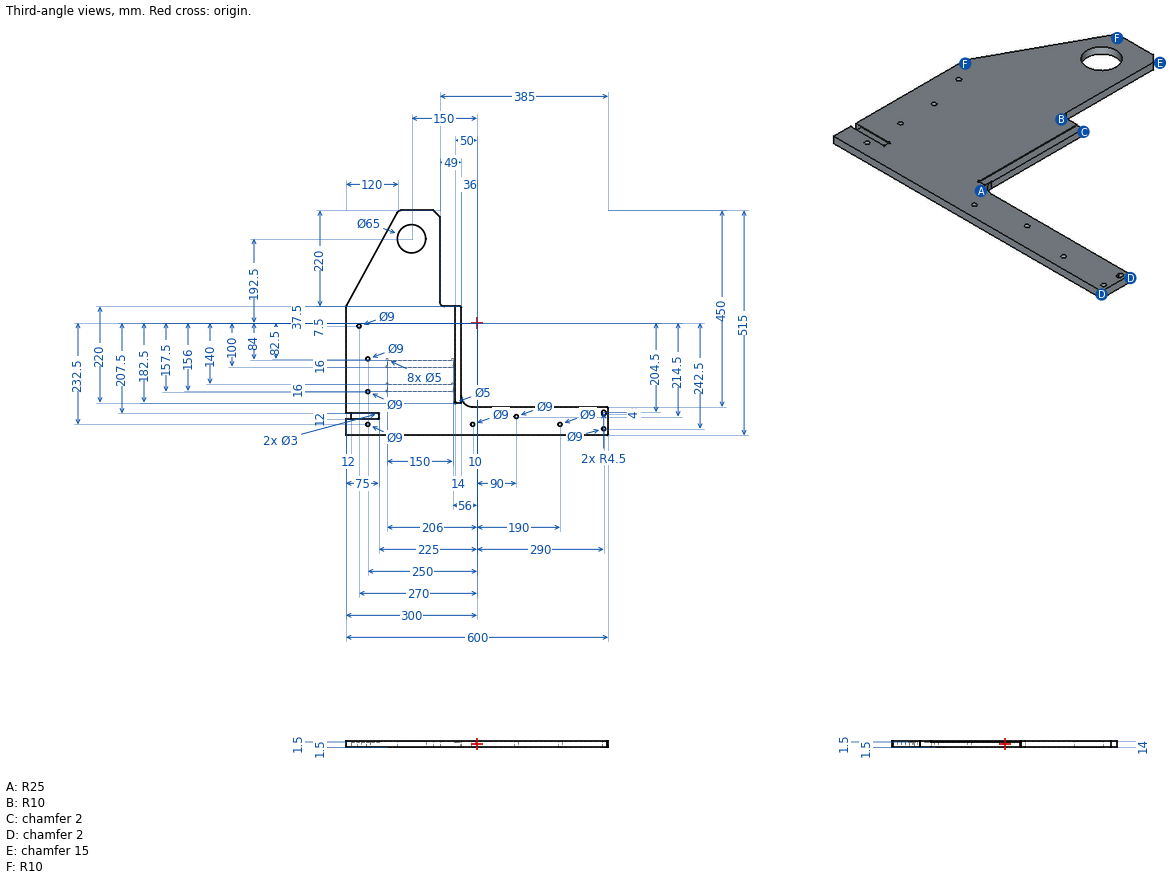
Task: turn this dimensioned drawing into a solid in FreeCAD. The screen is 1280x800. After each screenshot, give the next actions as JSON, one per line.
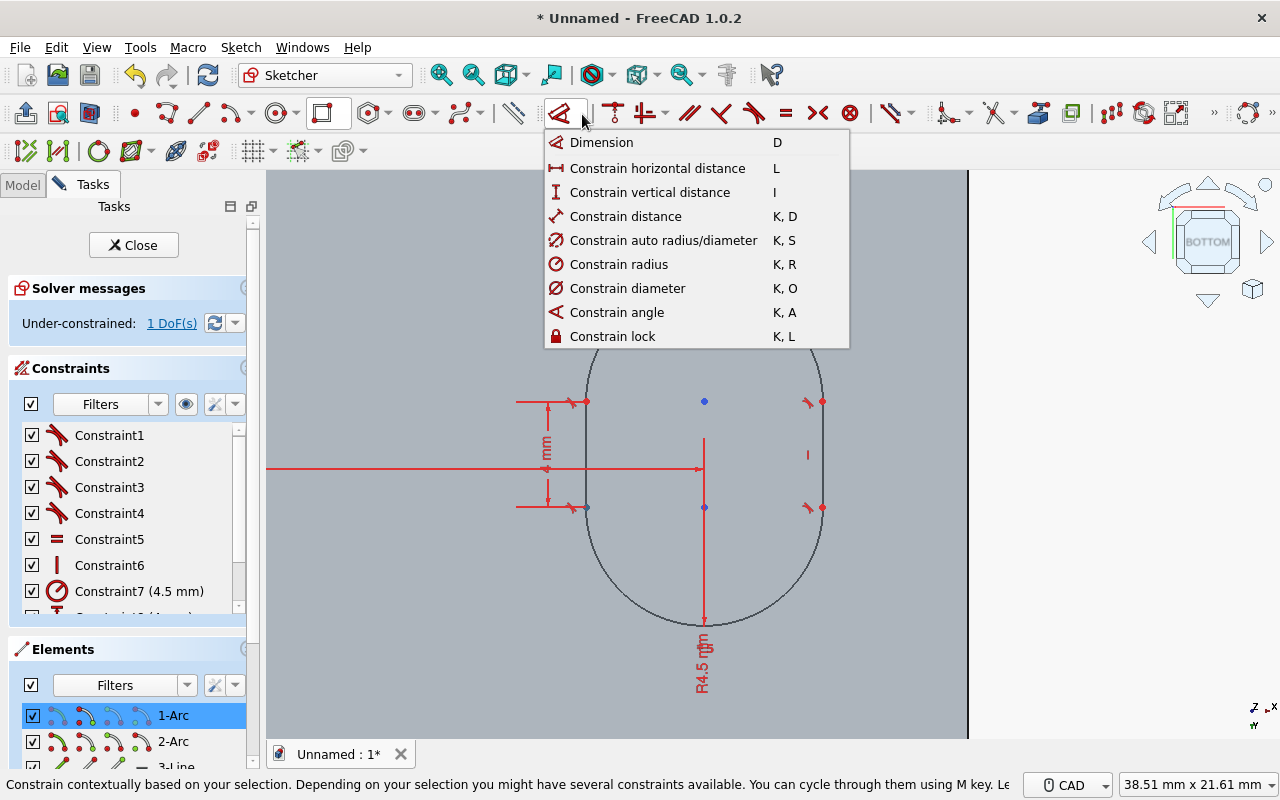
{"action": "left_click", "coordinate": [697, 192]}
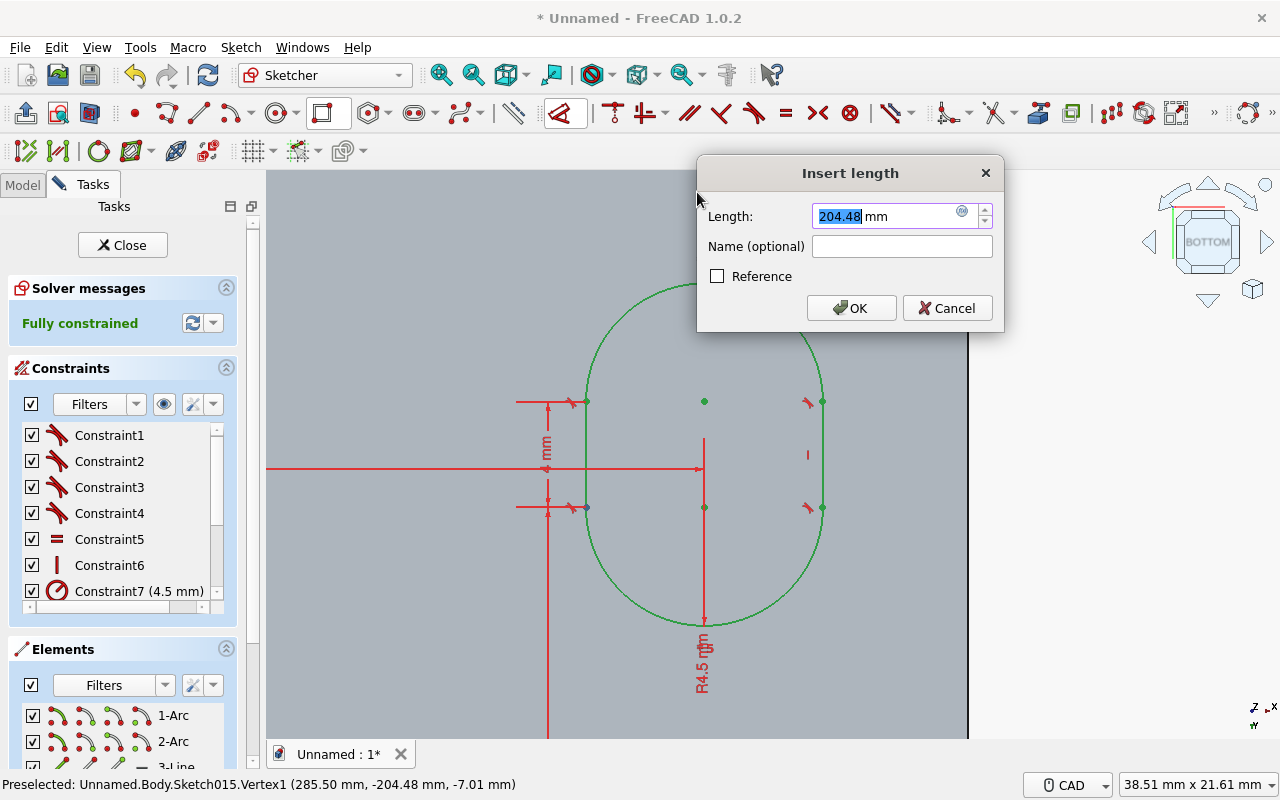
{"action": "type", "text": "204.5"}
{"action": "key", "text": "Return"}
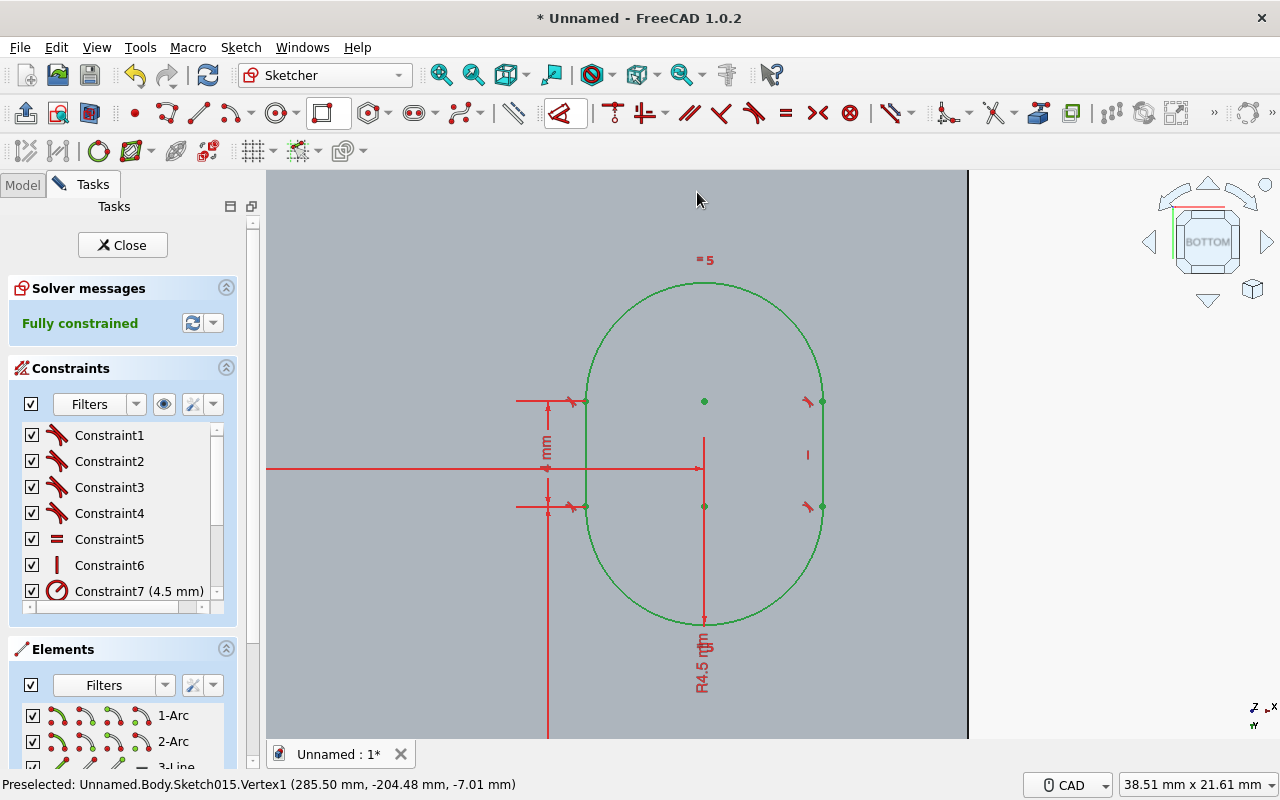
{"action": "left_click", "coordinate": [123, 245]}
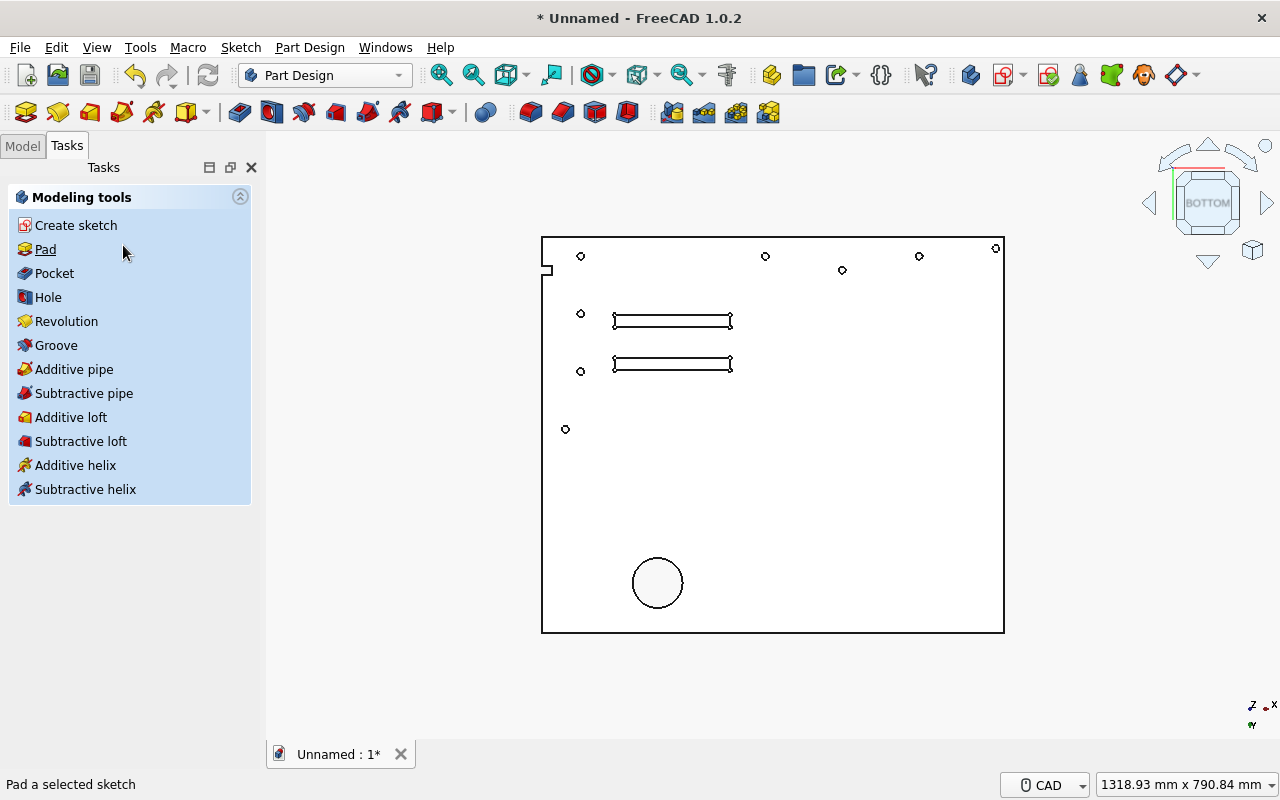
{"action": "left_click", "coordinate": [240, 112]}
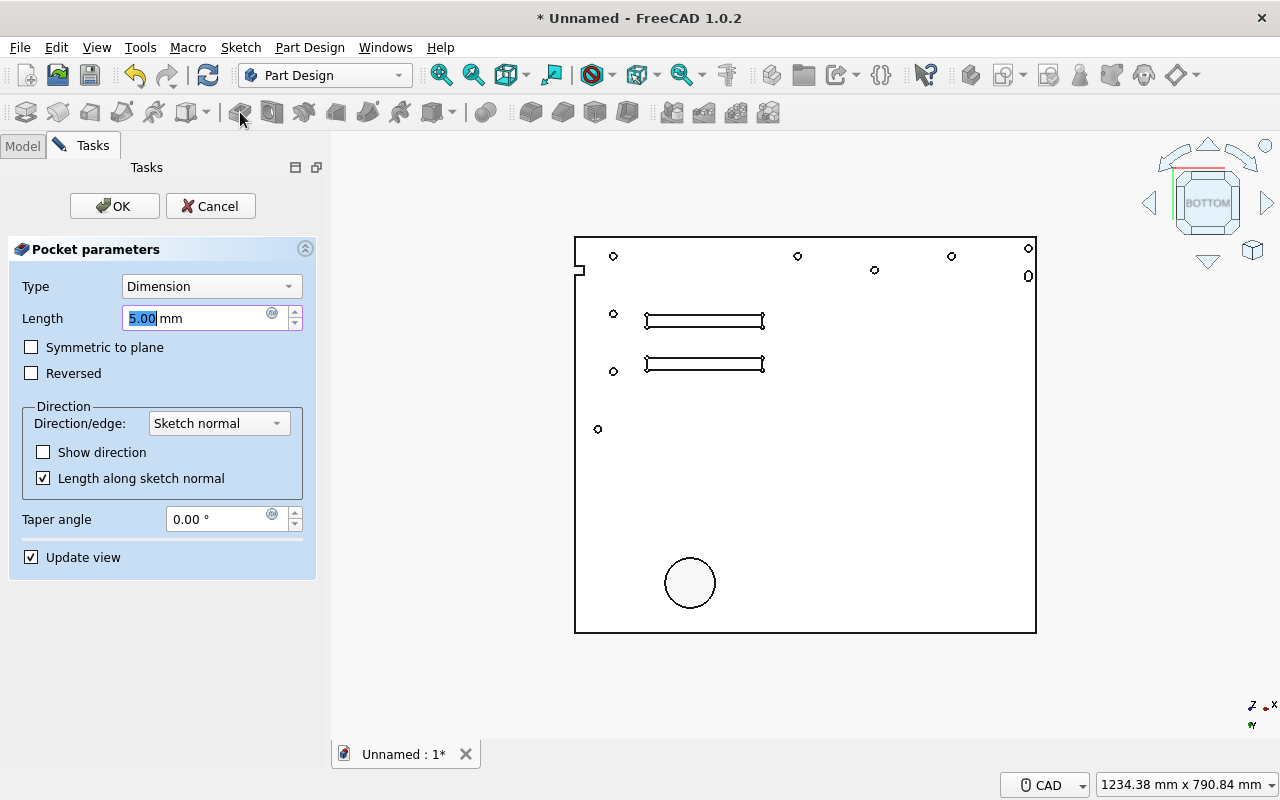
{"action": "left_click", "coordinate": [212, 286]}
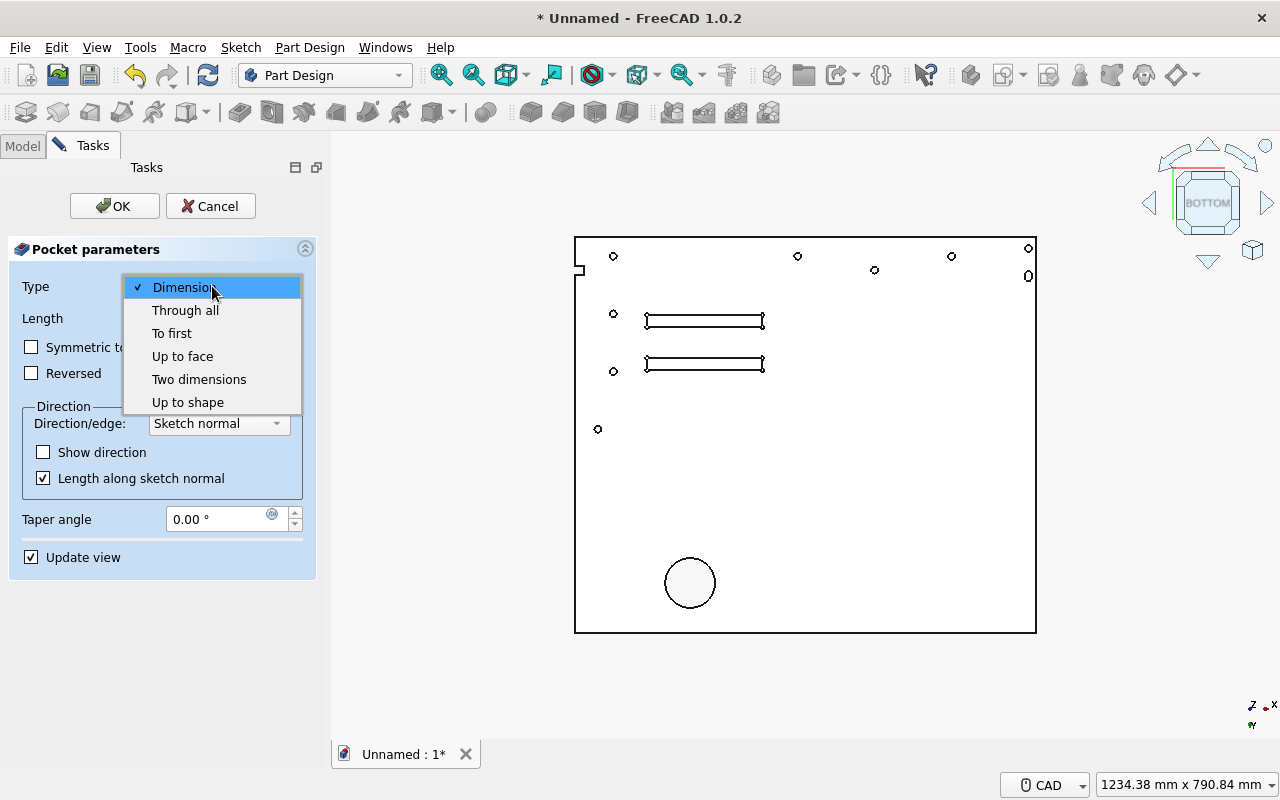
{"action": "left_click", "coordinate": [212, 334]}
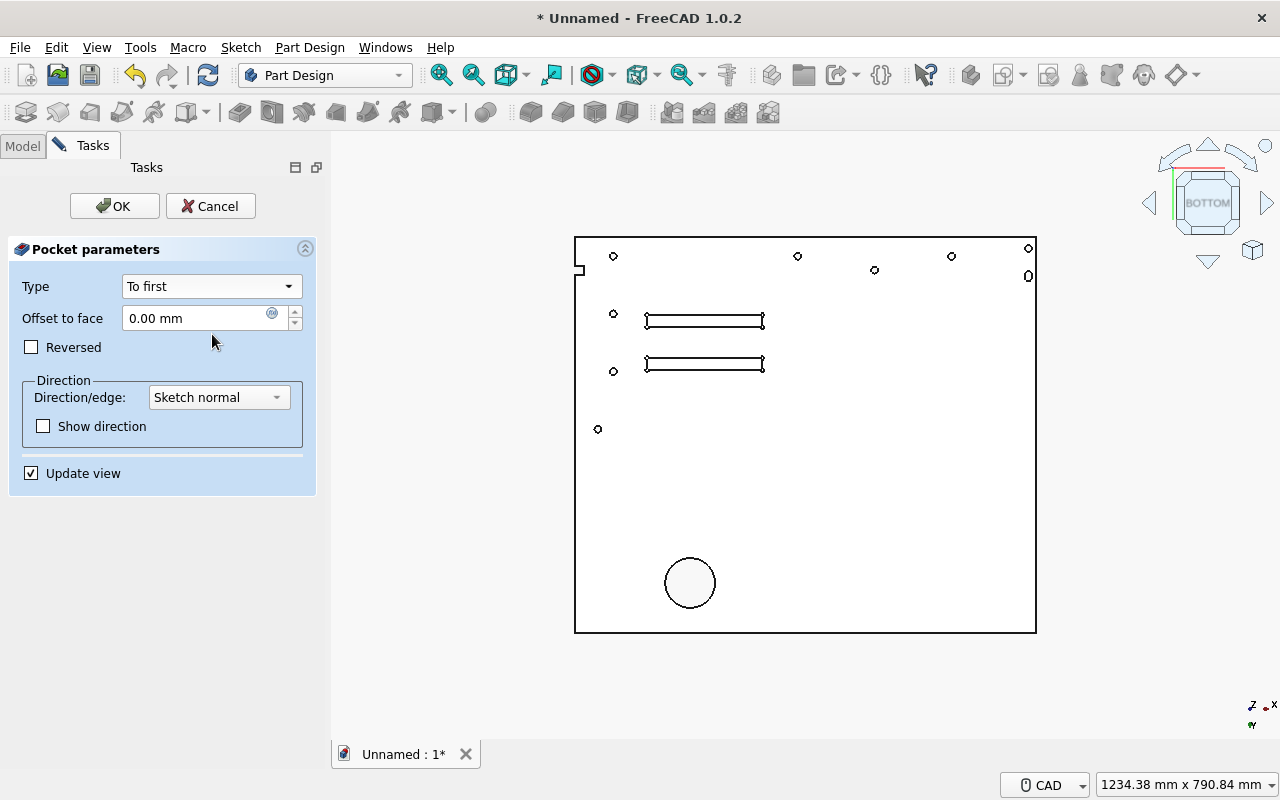
{"action": "left_click", "coordinate": [115, 206]}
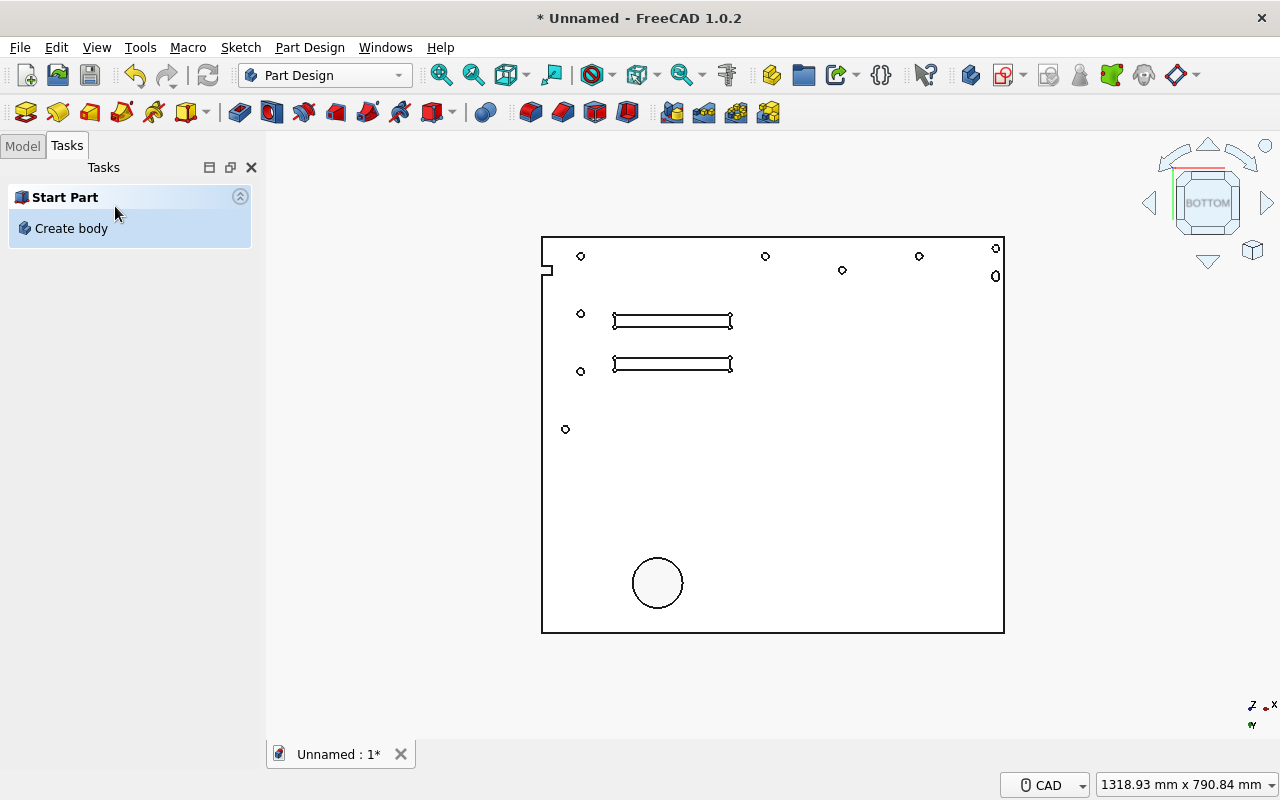
{"action": "left_click", "coordinate": [839, 491]}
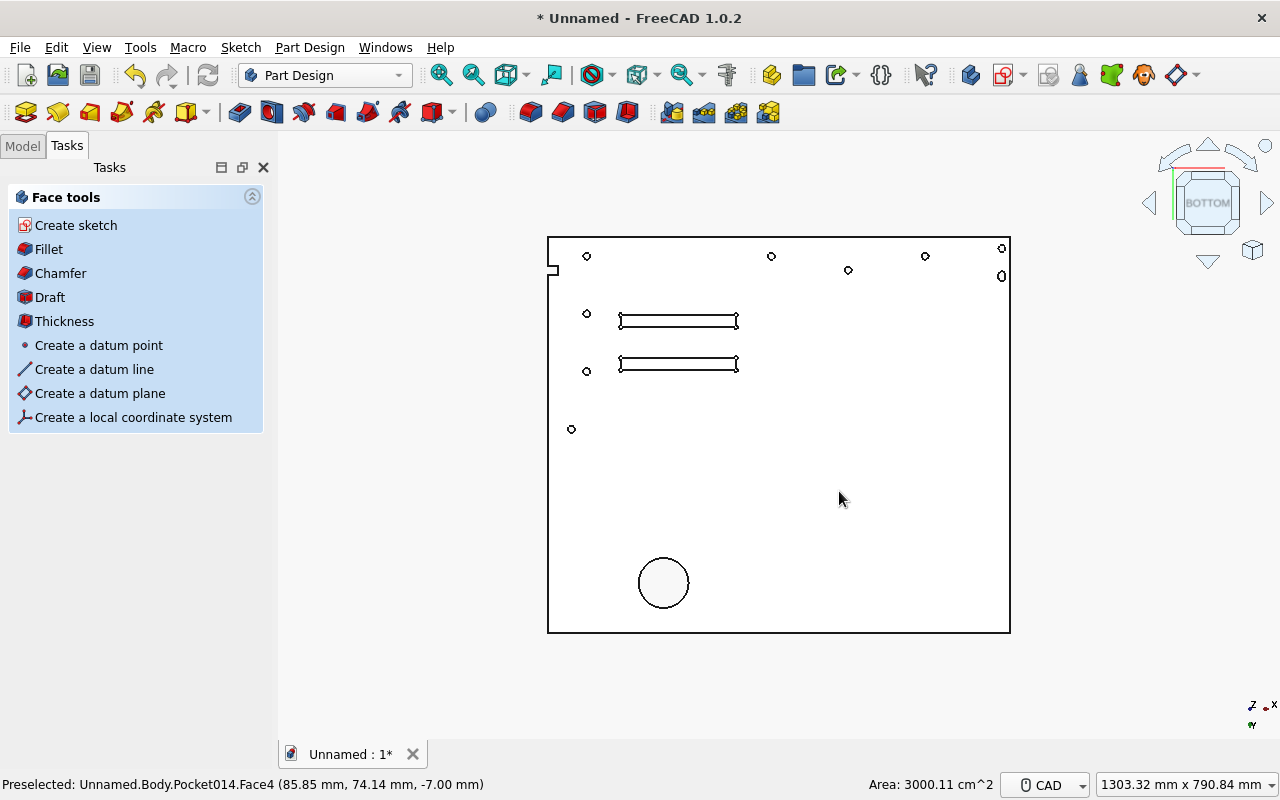
{"action": "left_click", "coordinate": [1004, 76]}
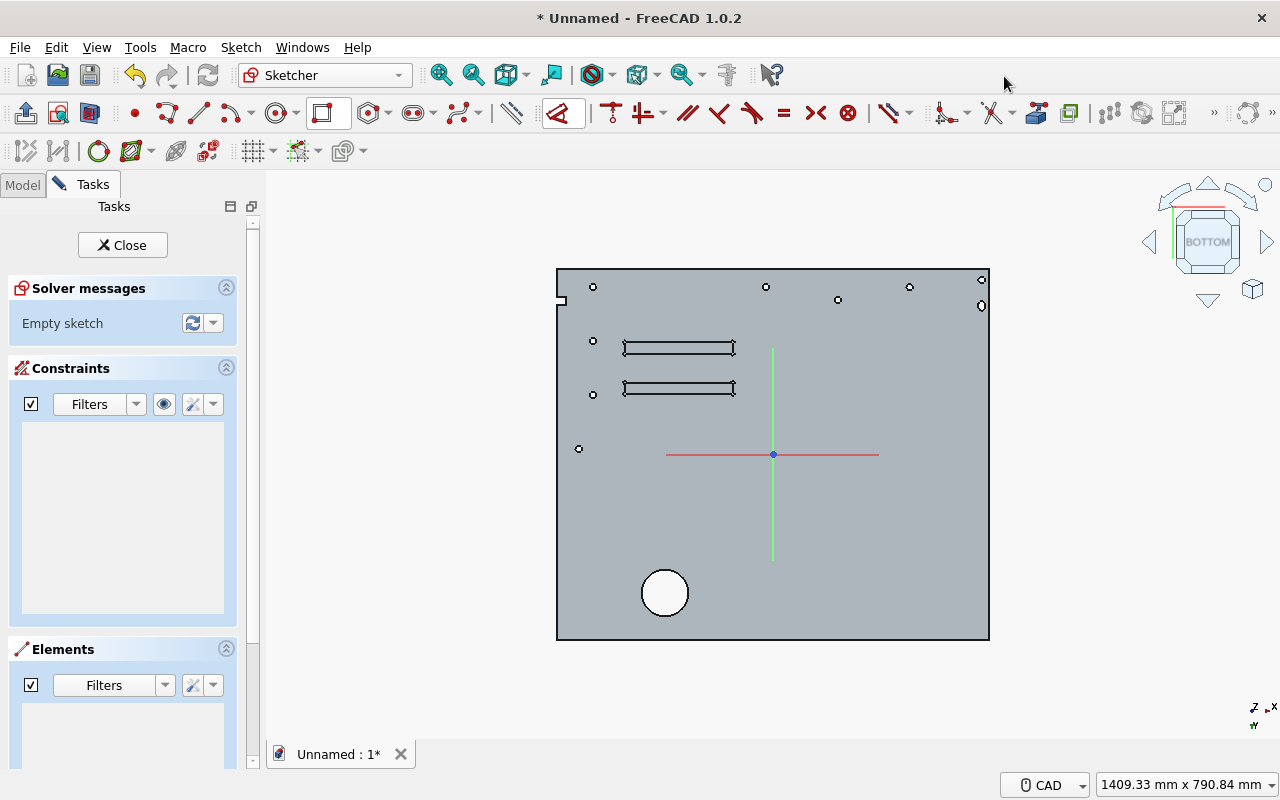
{"action": "left_click", "coordinate": [168, 114]}